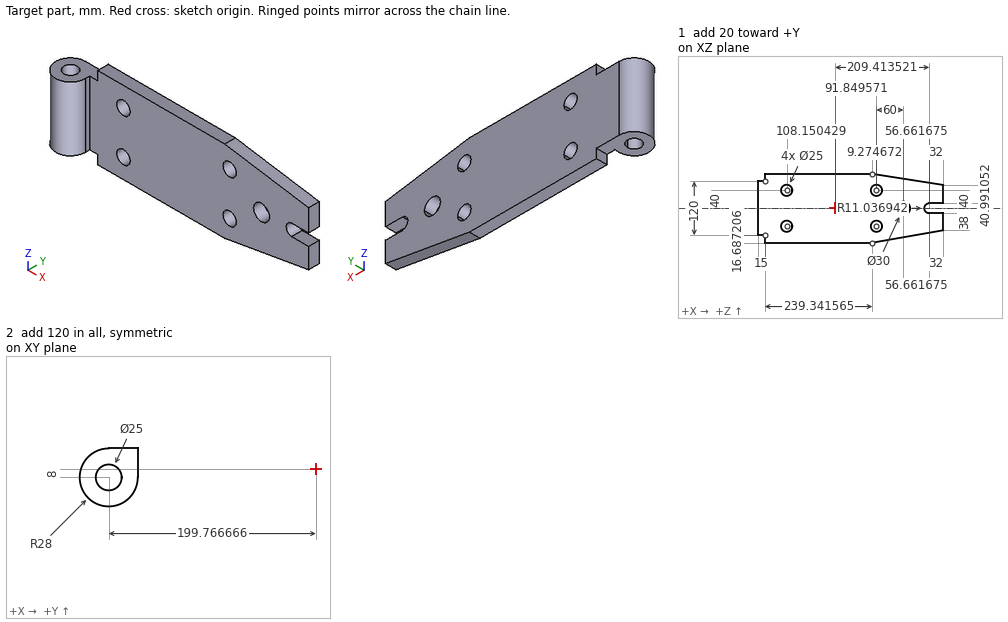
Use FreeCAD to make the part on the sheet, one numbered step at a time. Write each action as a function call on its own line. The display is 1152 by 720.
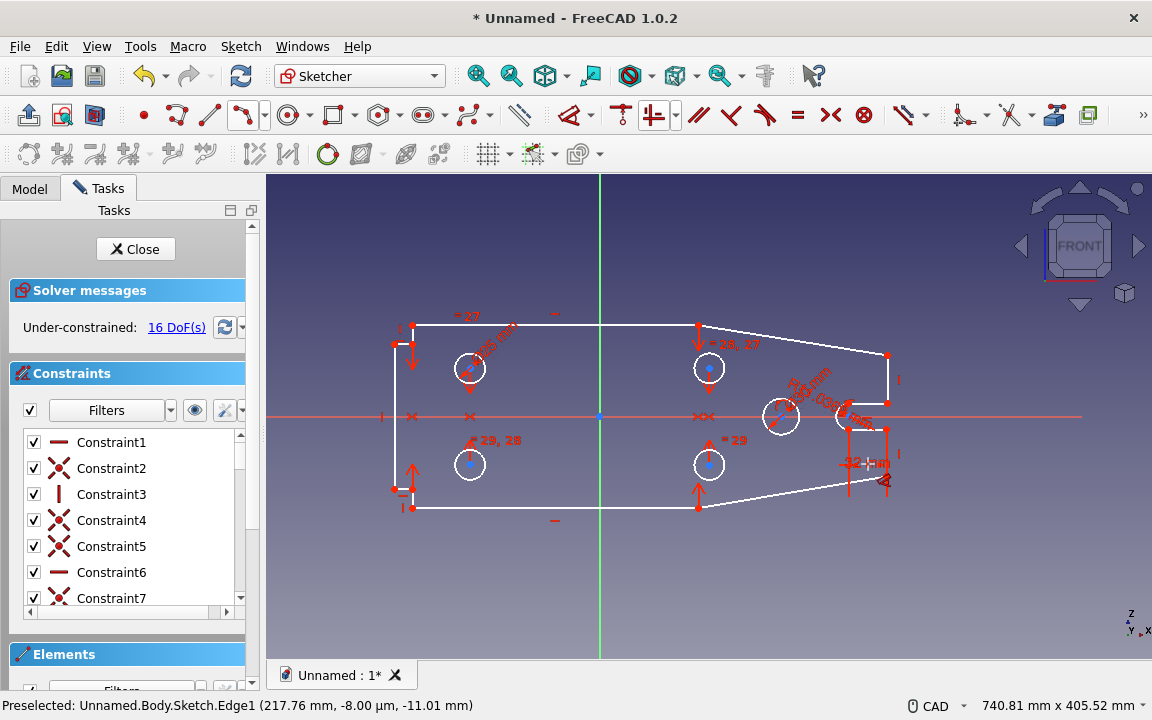
click(887, 444)
click(921, 442)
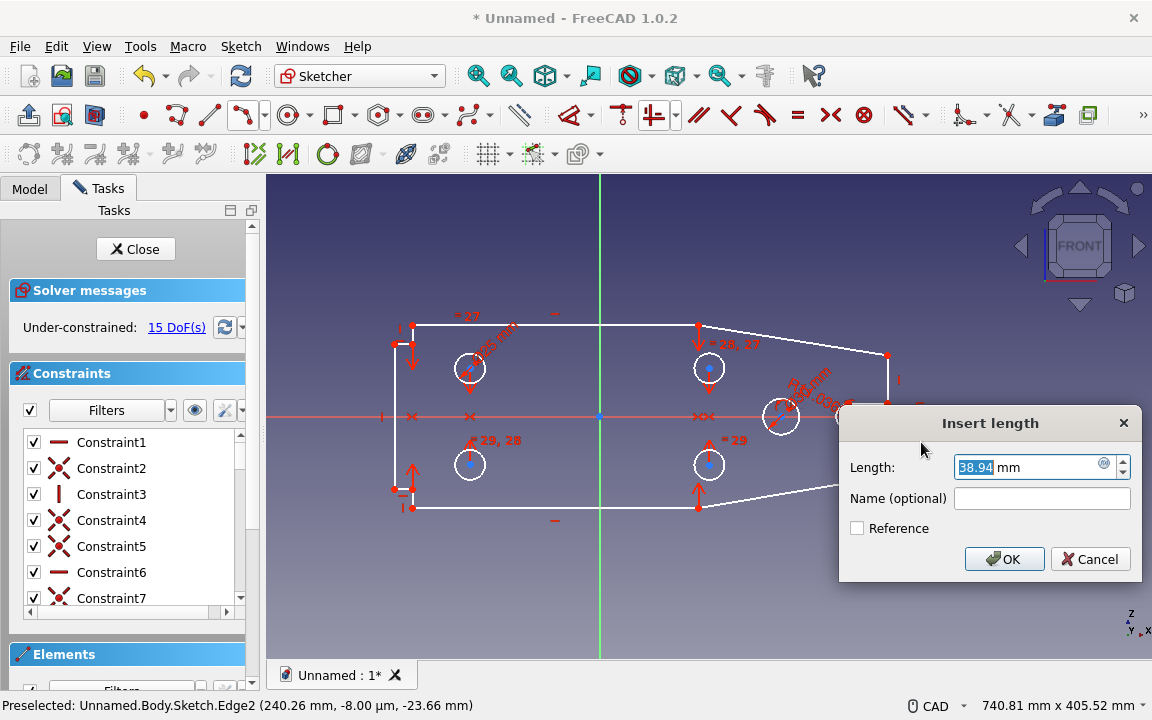
text(38)
key(Return)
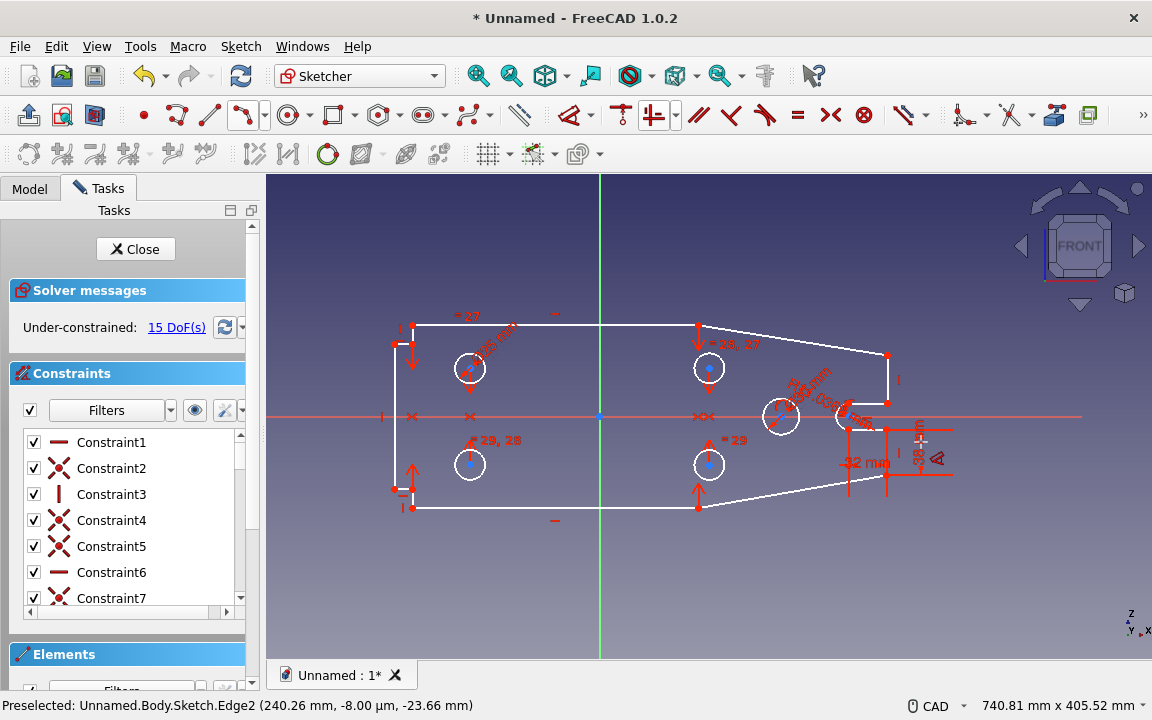
scroll(404, 489, up, 4)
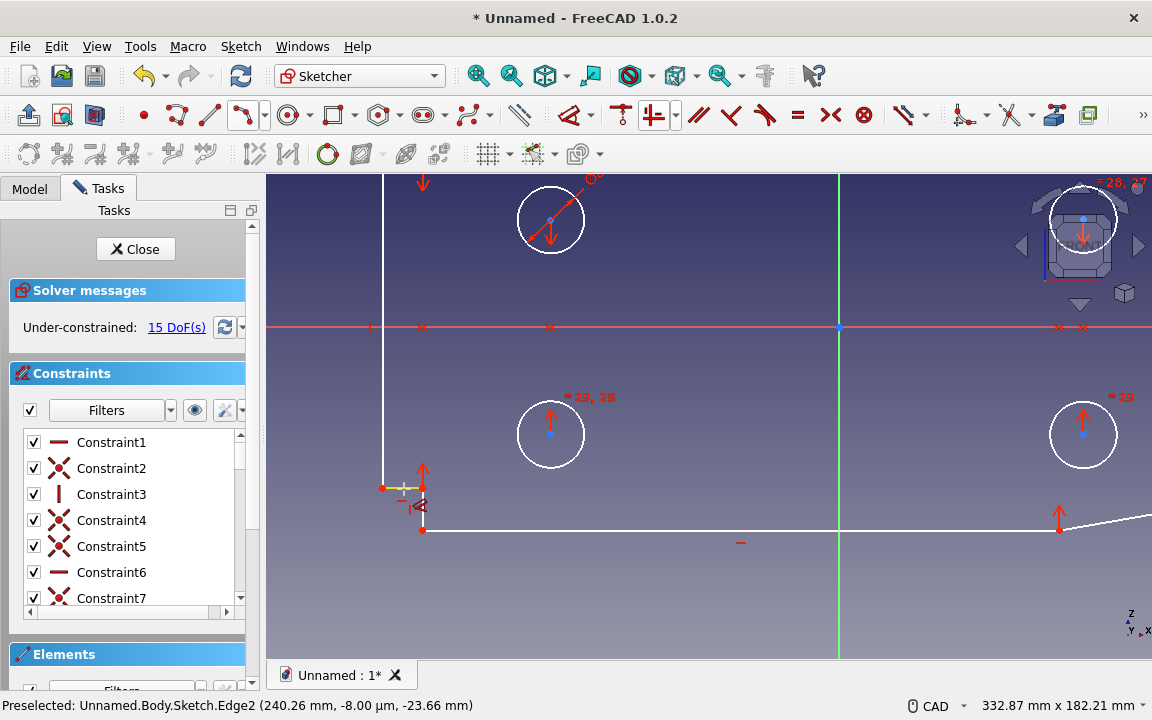
click(403, 488)
click(403, 522)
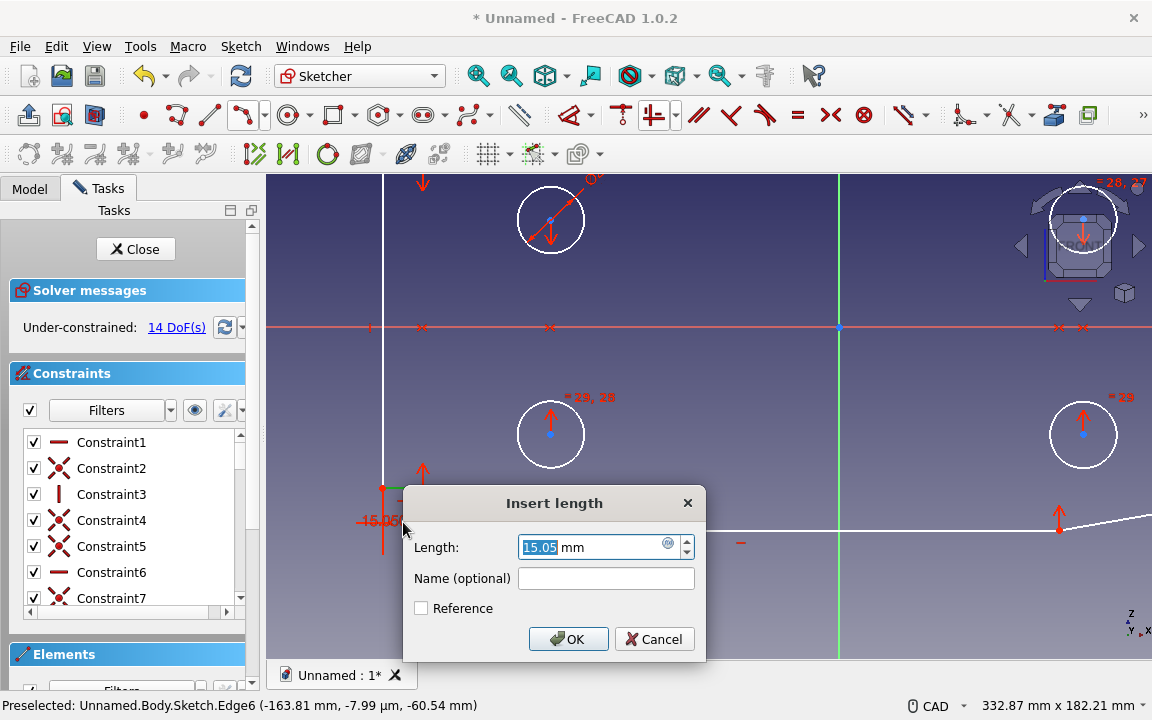
text(15)
key(Return)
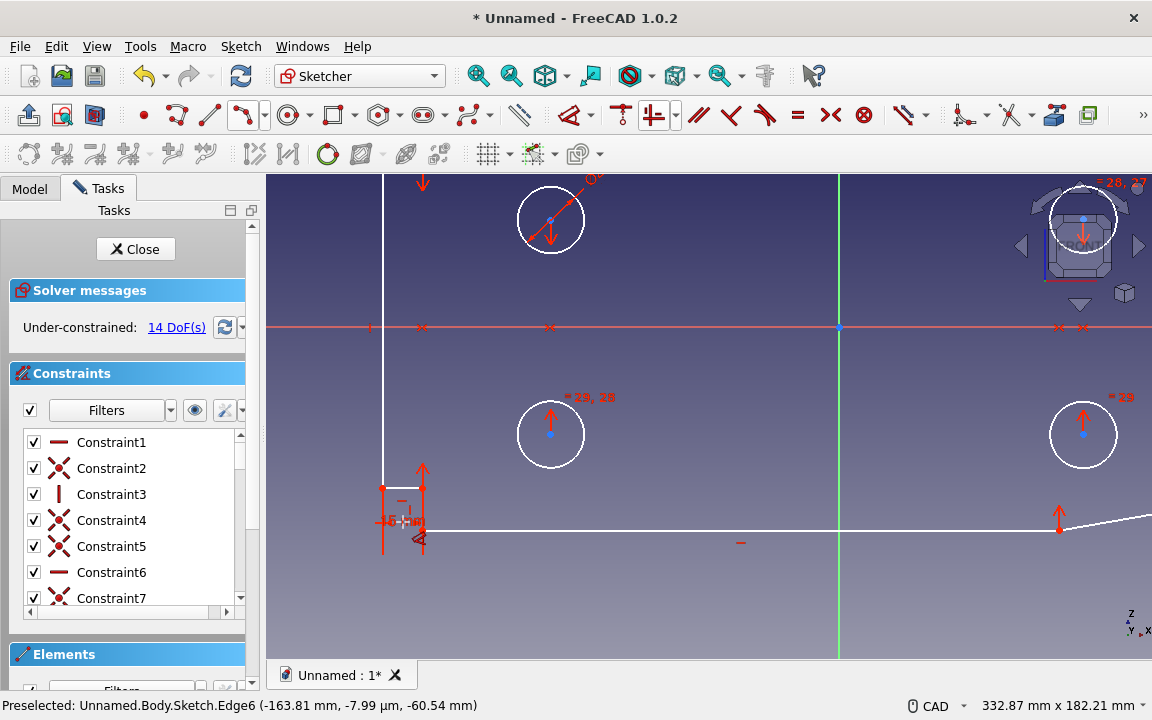
scroll(404, 489, down, 4)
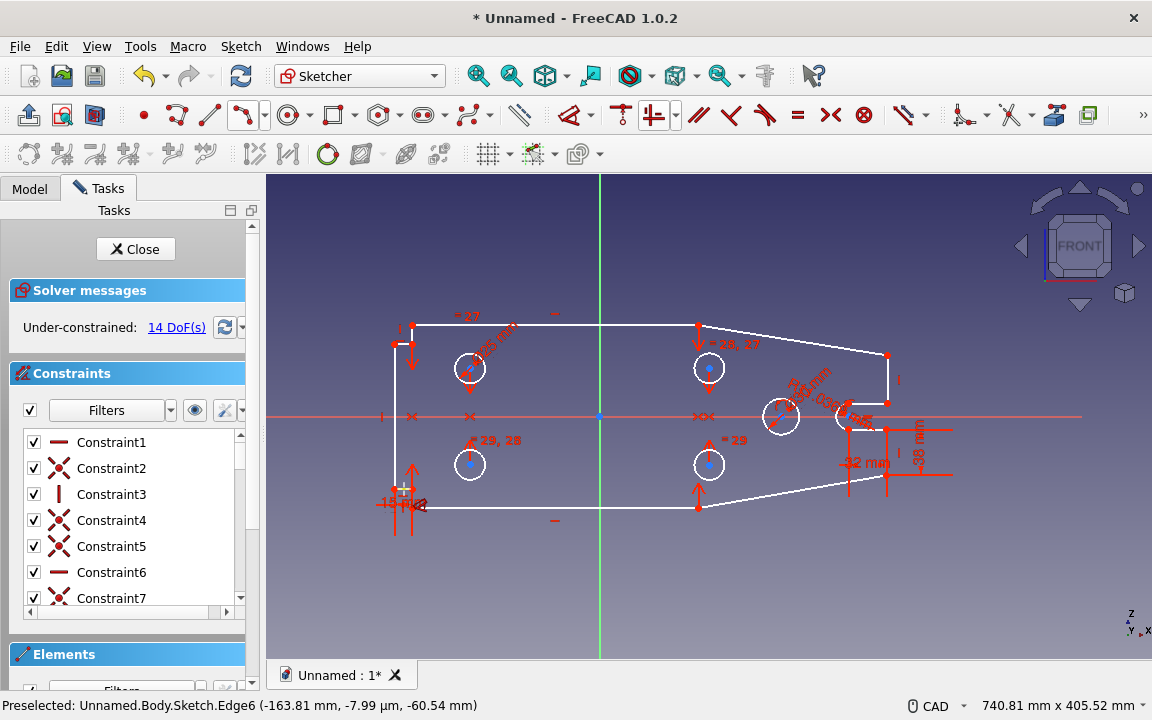
click(876, 404)
click(868, 322)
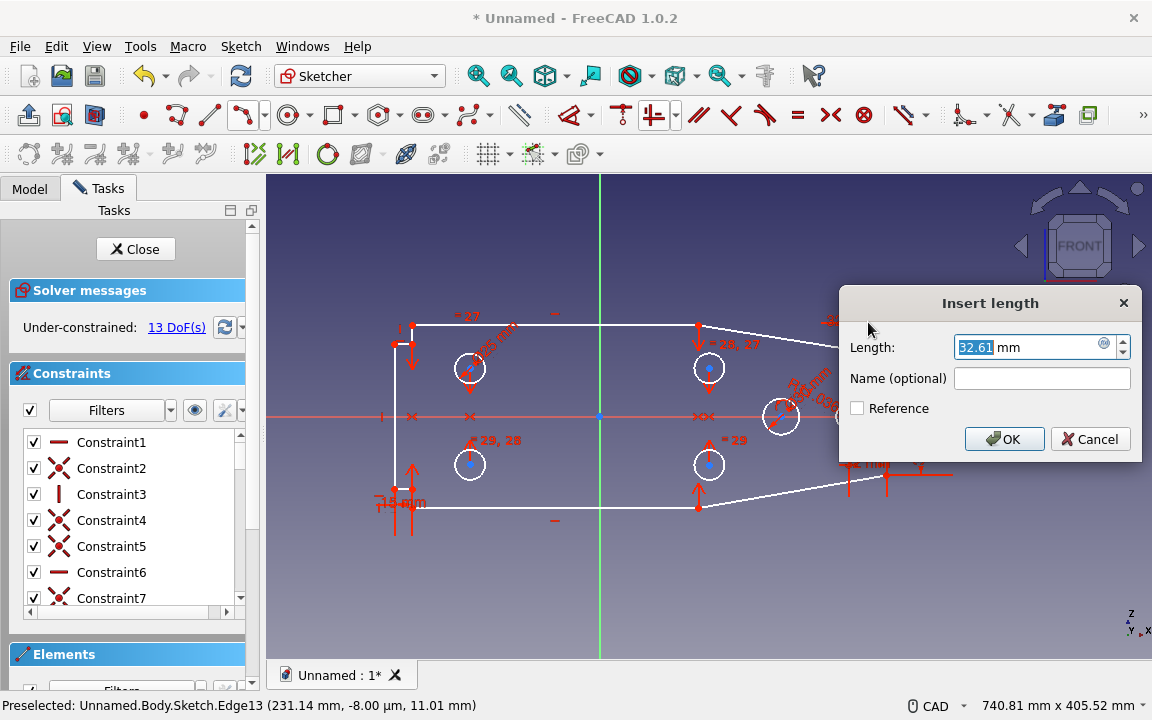
text(32)
key(Return)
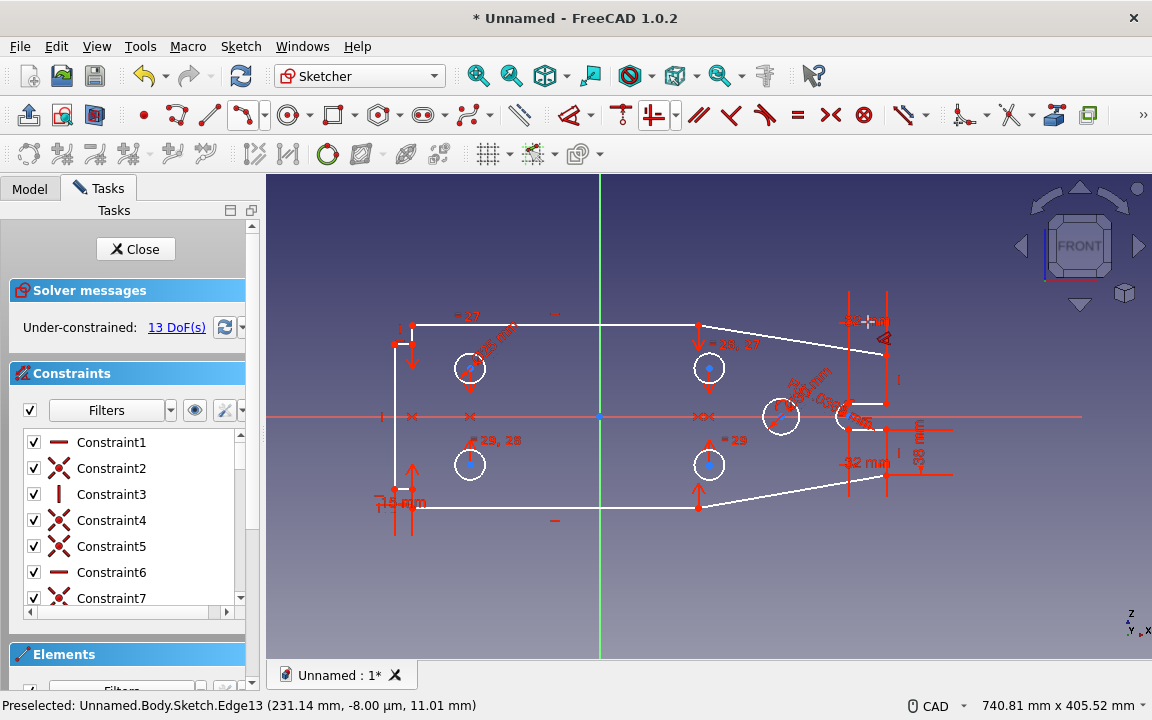
click(470, 369)
click(436, 393)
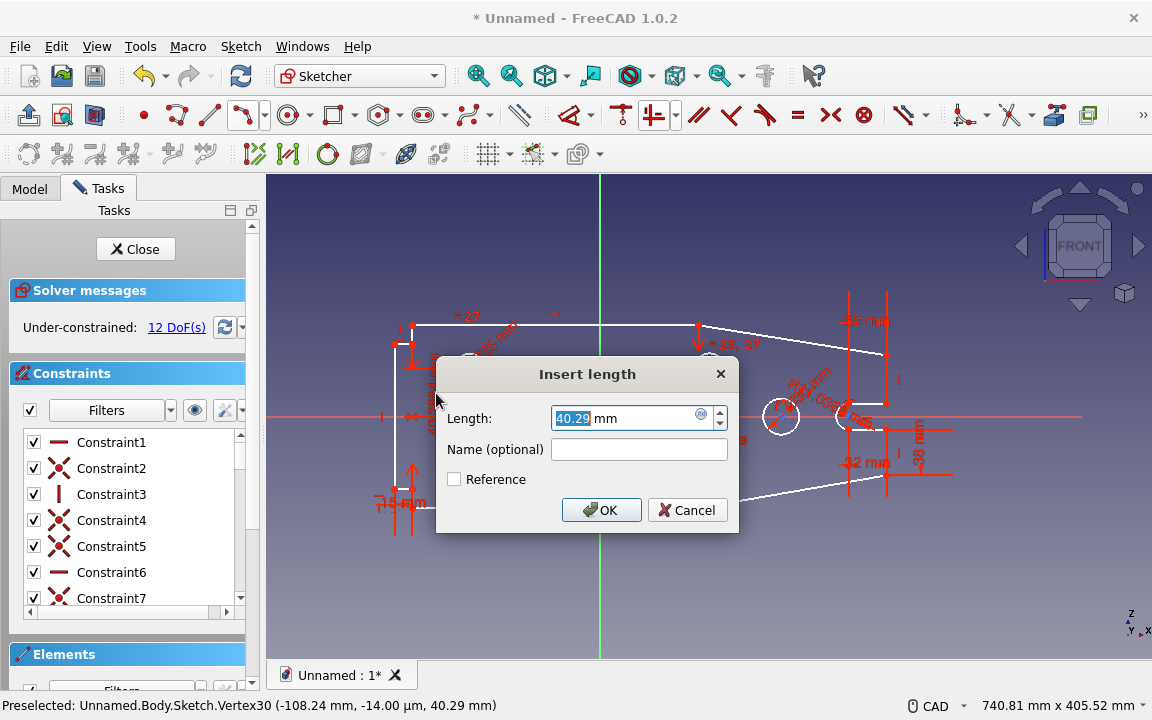
text(40)
key(Return)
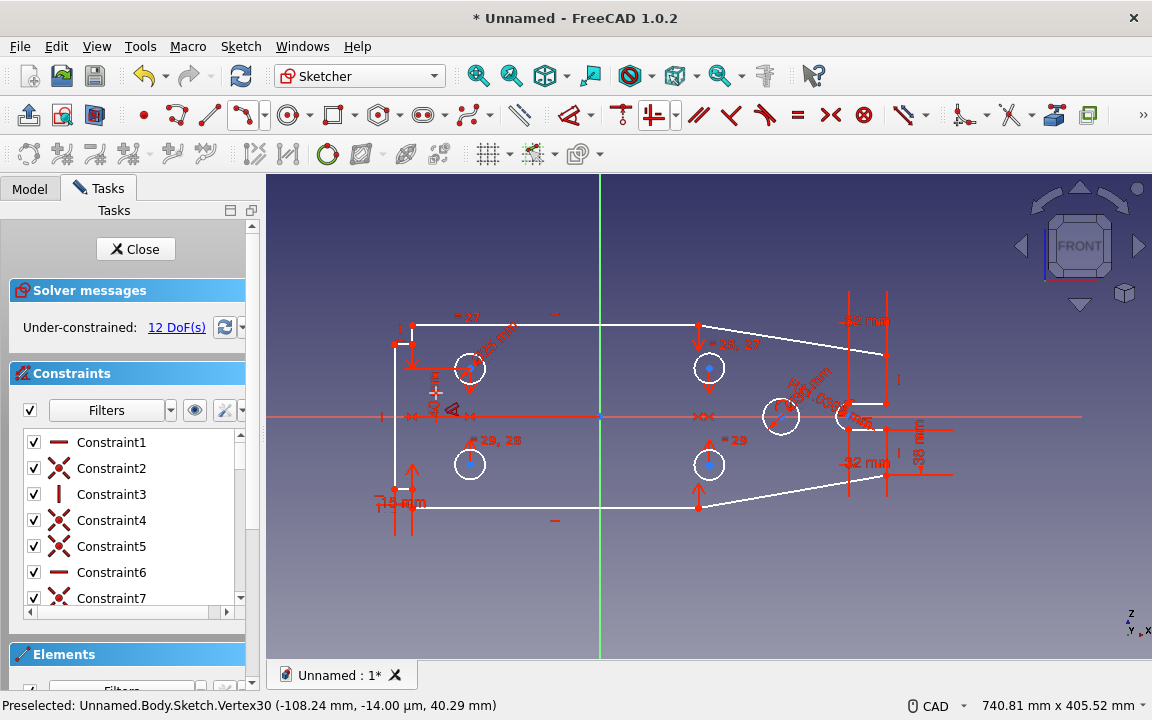
click(709, 368)
click(566, 393)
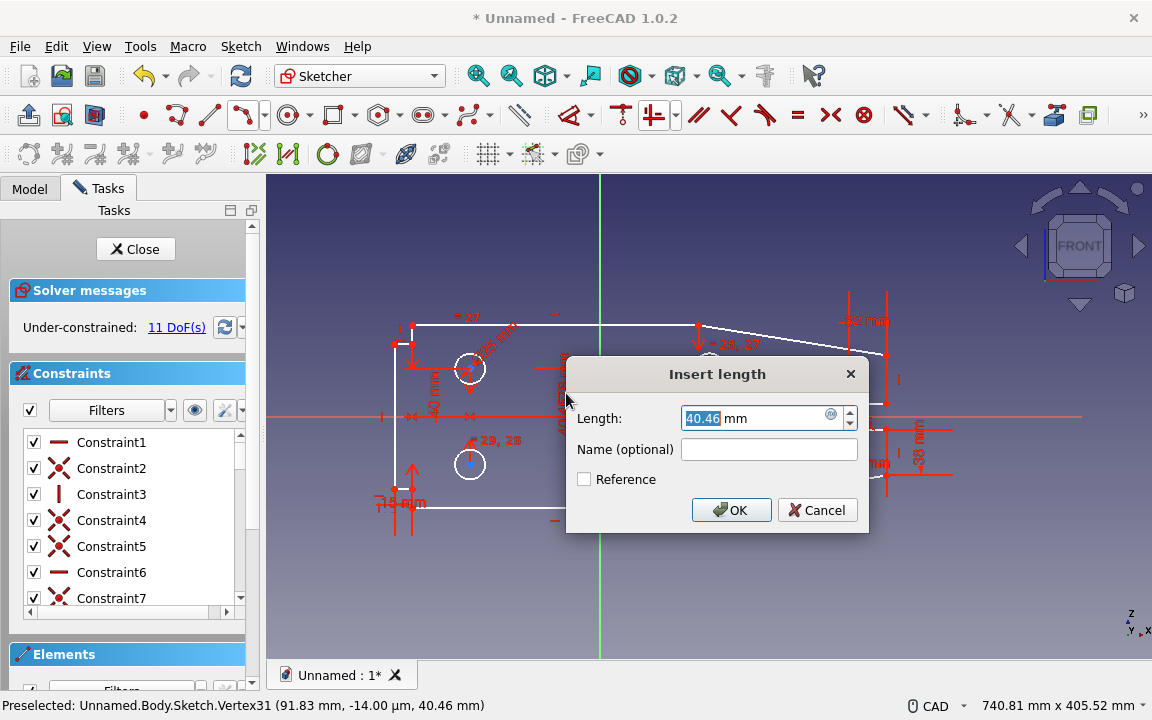
text(40)
key(Return)